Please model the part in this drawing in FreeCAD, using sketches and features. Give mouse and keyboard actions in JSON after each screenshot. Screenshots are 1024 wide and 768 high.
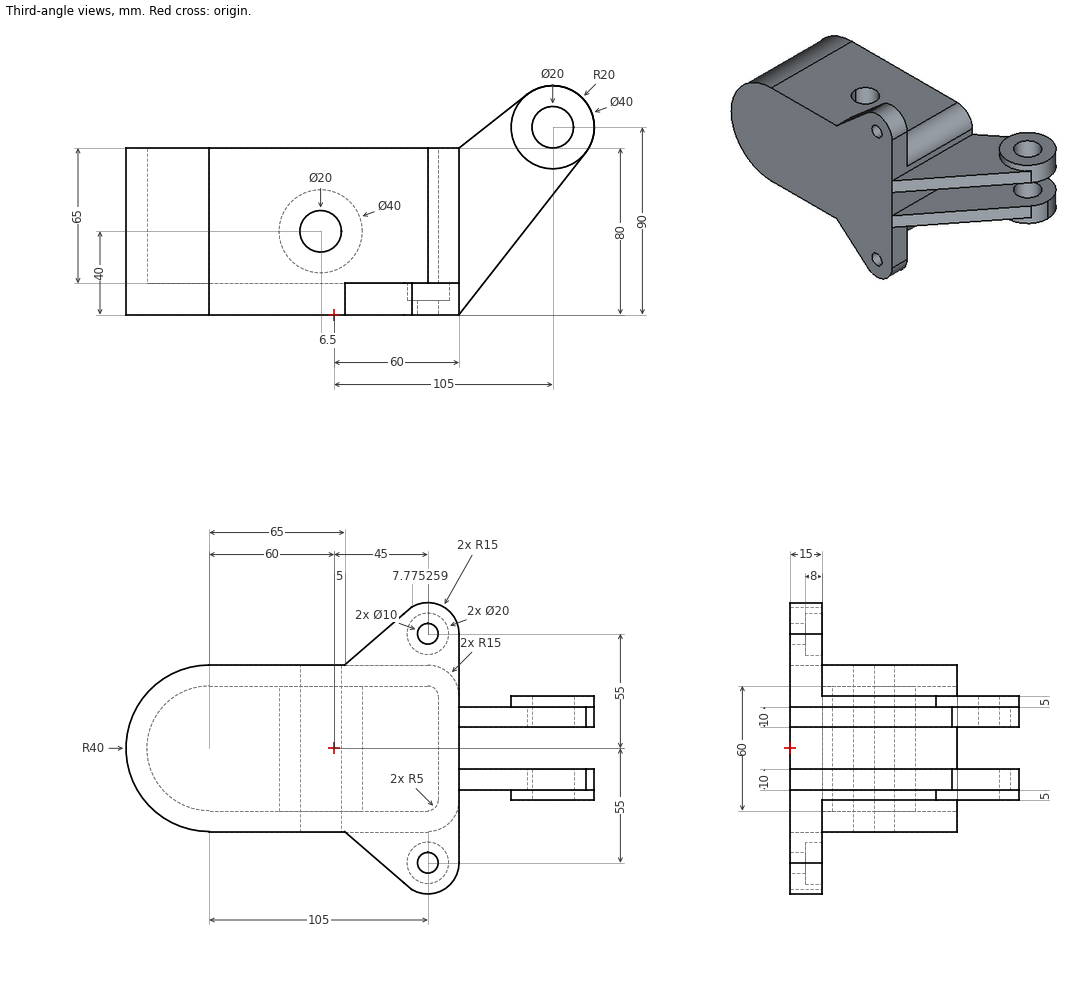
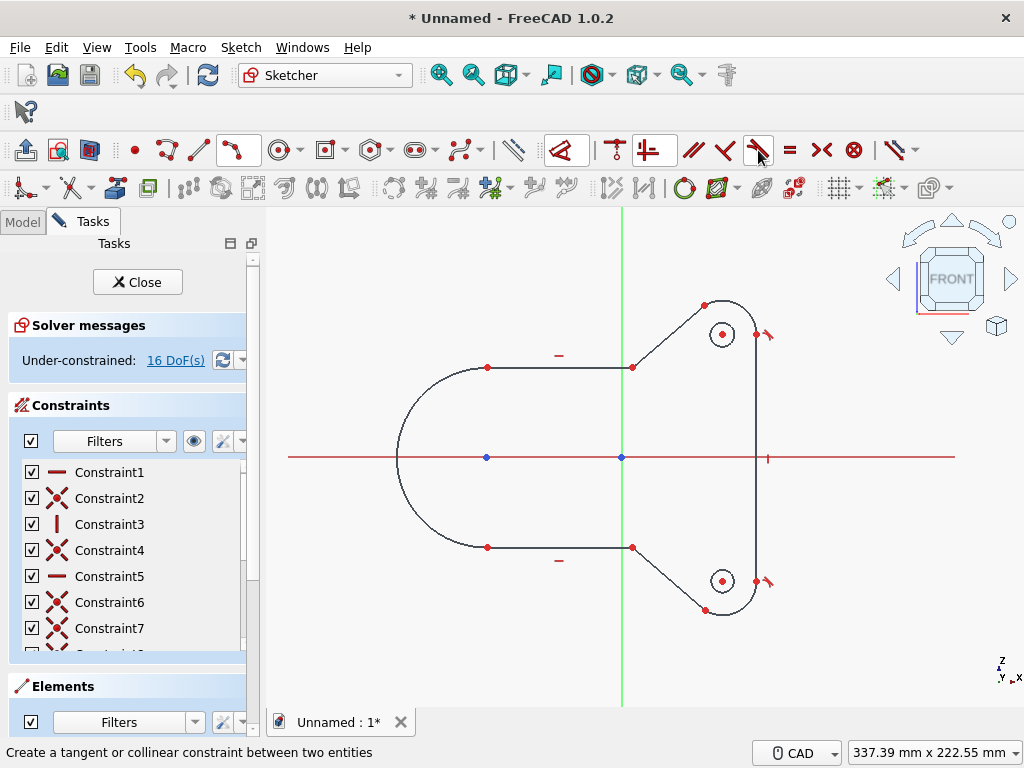
{"action": "left_click", "coordinate": [750, 315]}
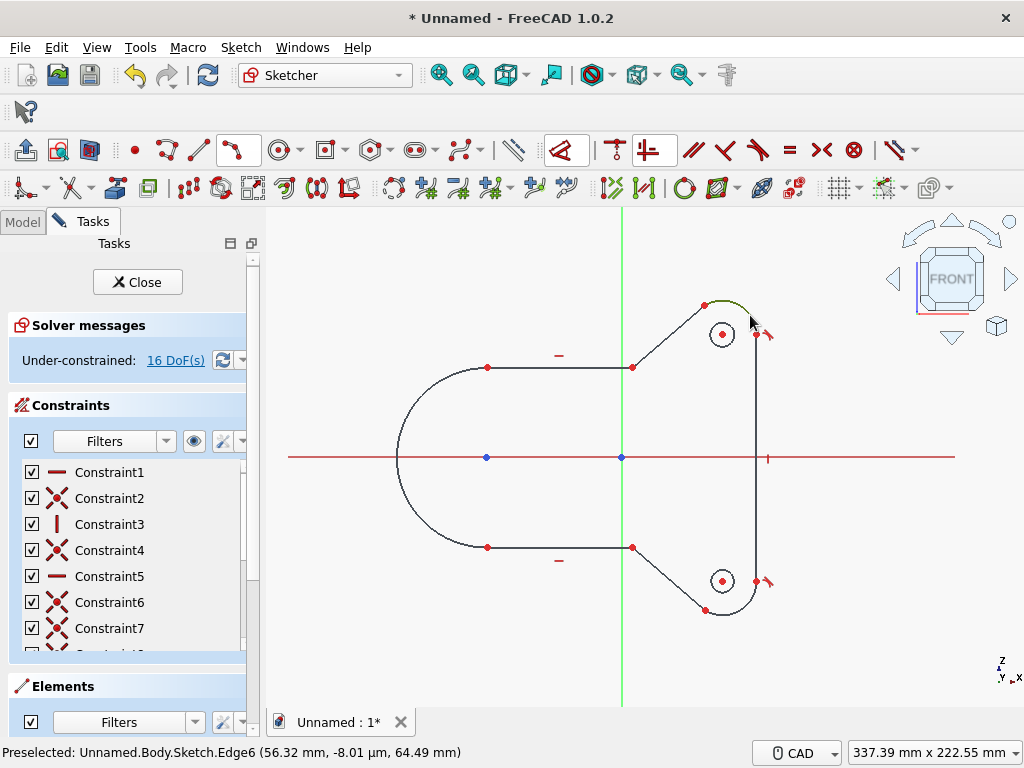
{"action": "left_click", "coordinate": [726, 615]}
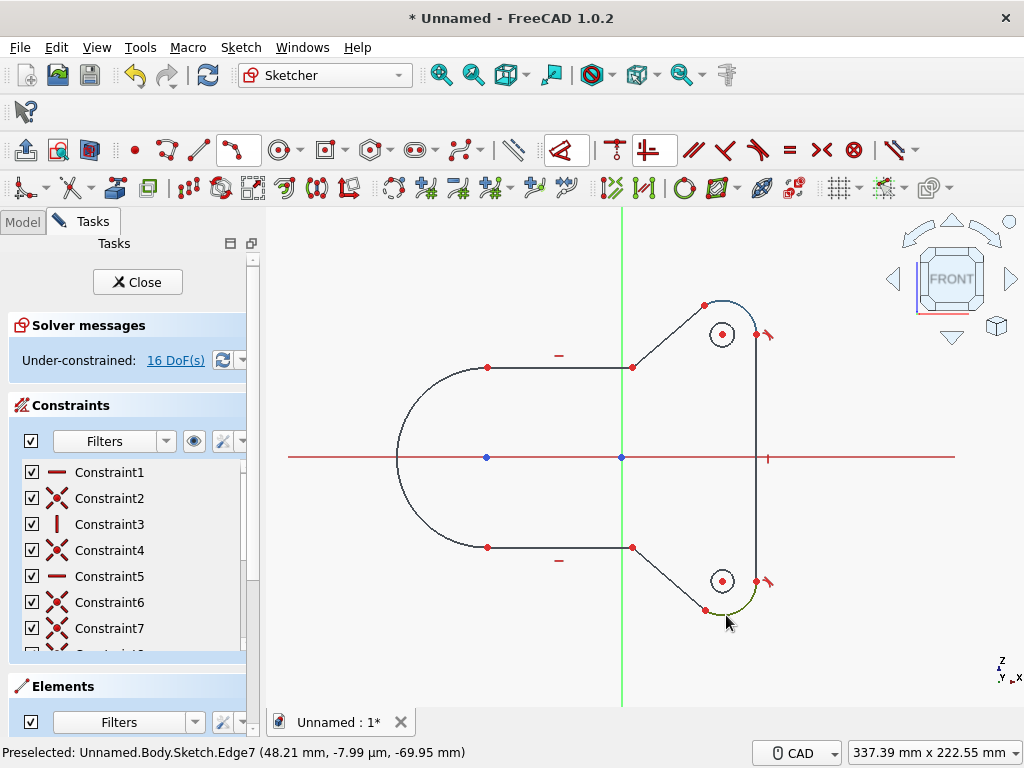
{"action": "left_click", "coordinate": [790, 150]}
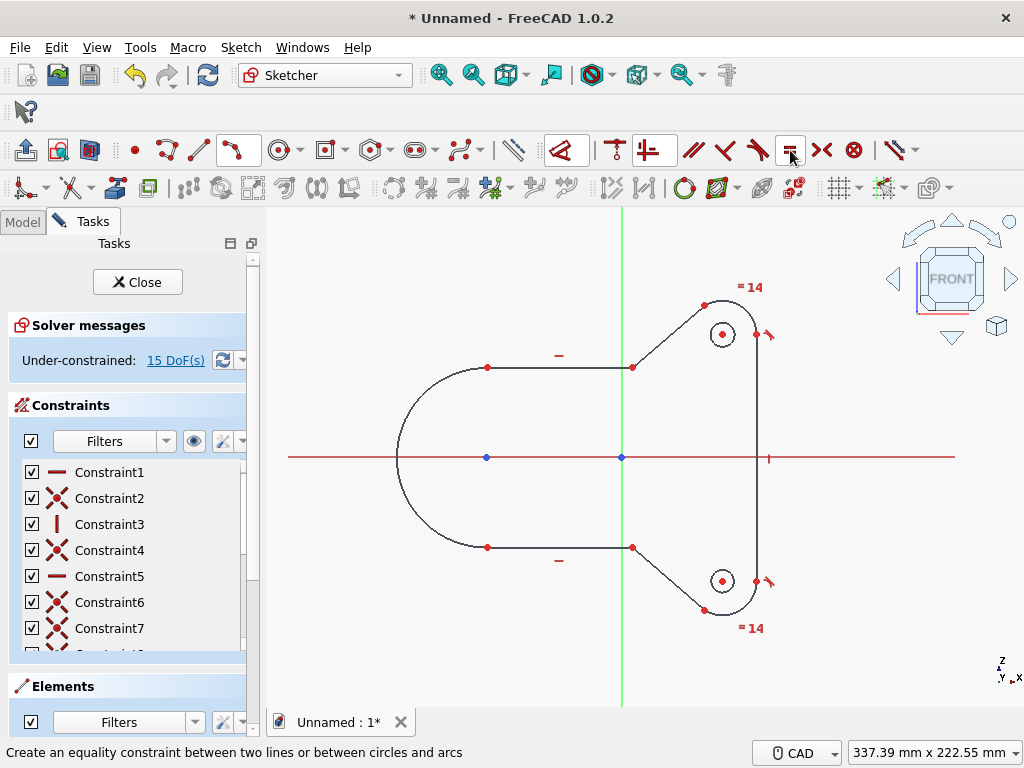
{"action": "left_click", "coordinate": [731, 326]}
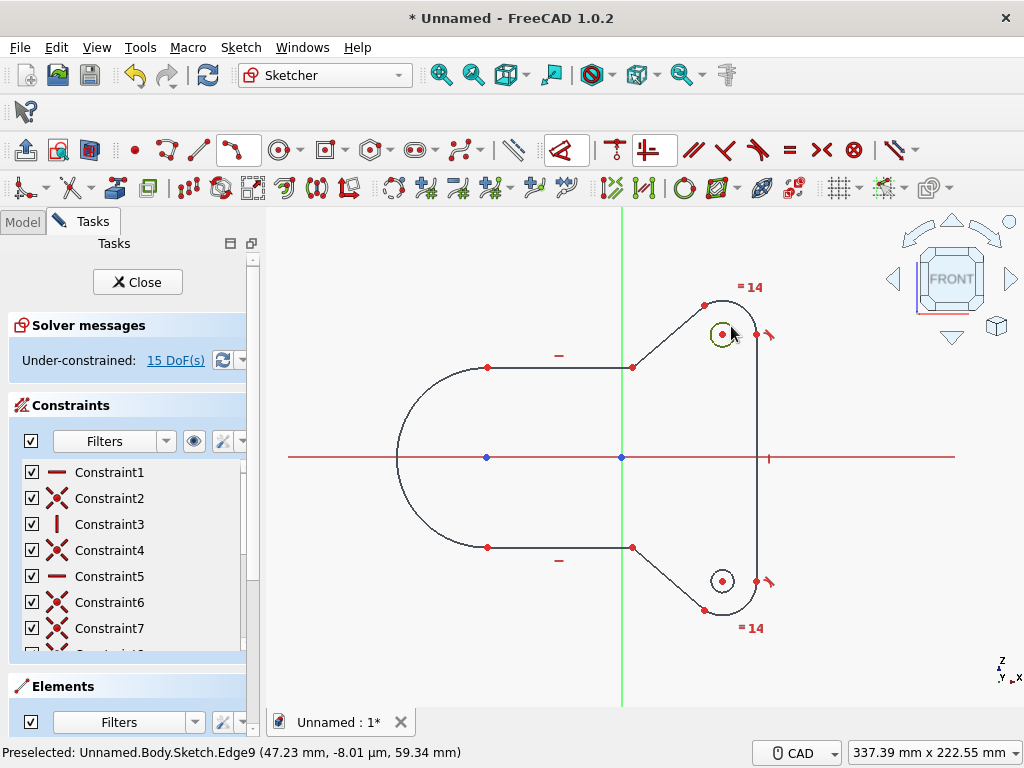
{"action": "scroll", "coordinate": [730, 573], "scroll_direction": "up", "scroll_amount": 2}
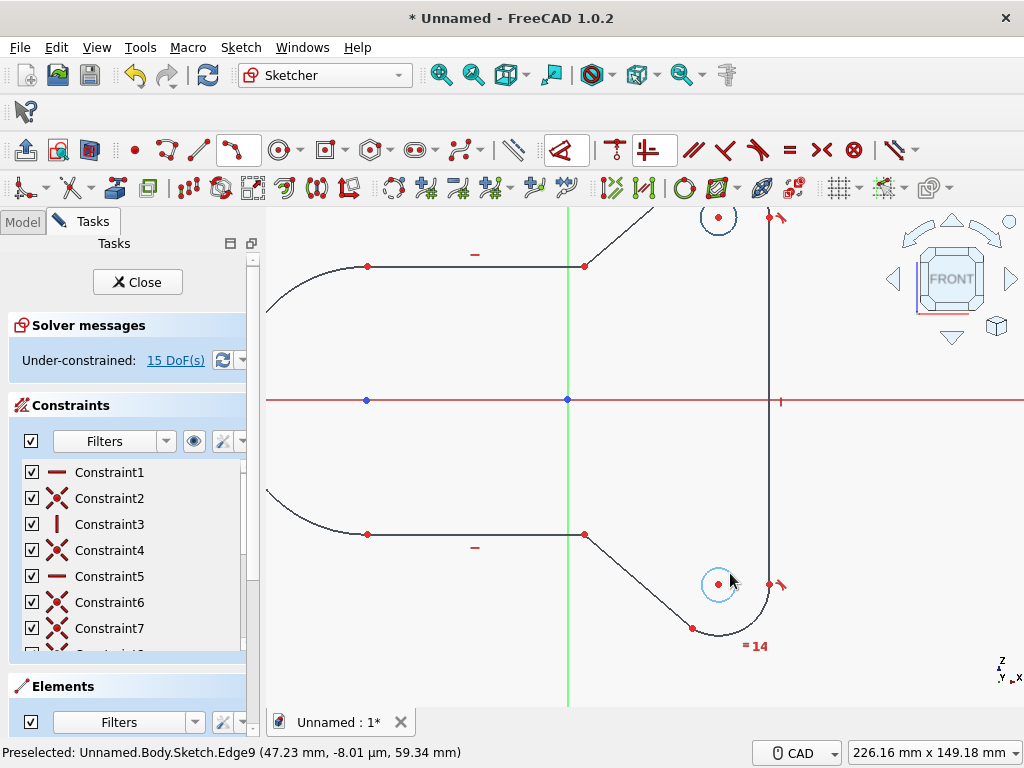
{"action": "left_click", "coordinate": [730, 573]}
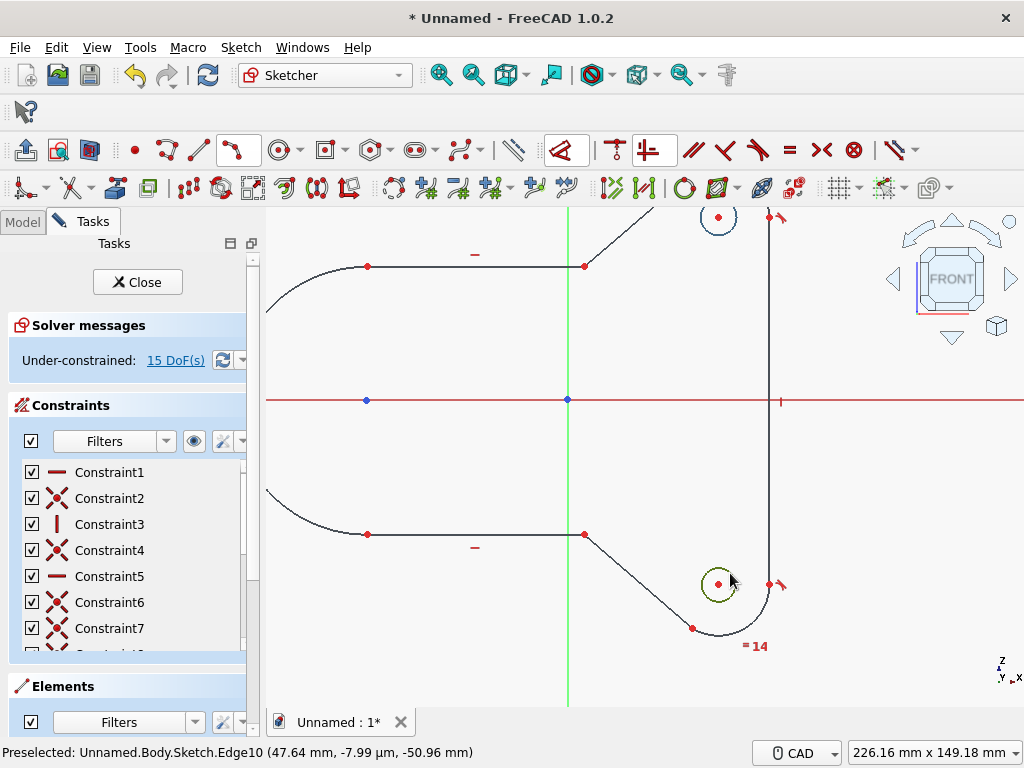
{"action": "left_click", "coordinate": [790, 150]}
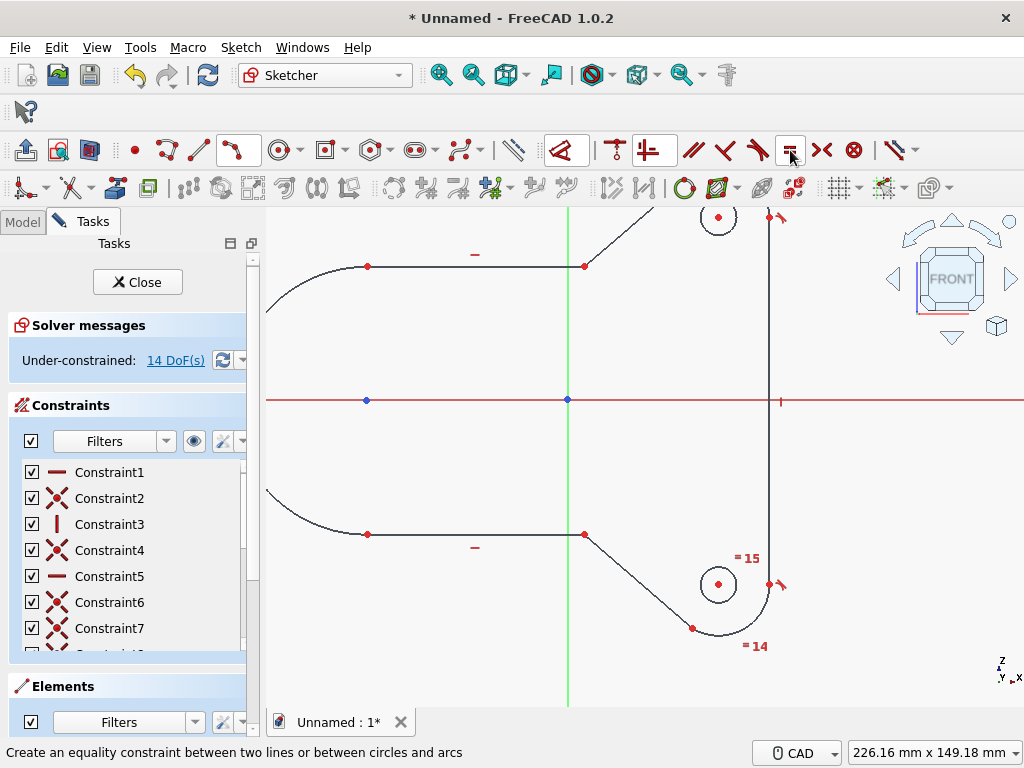
{"action": "left_click", "coordinate": [367, 401]}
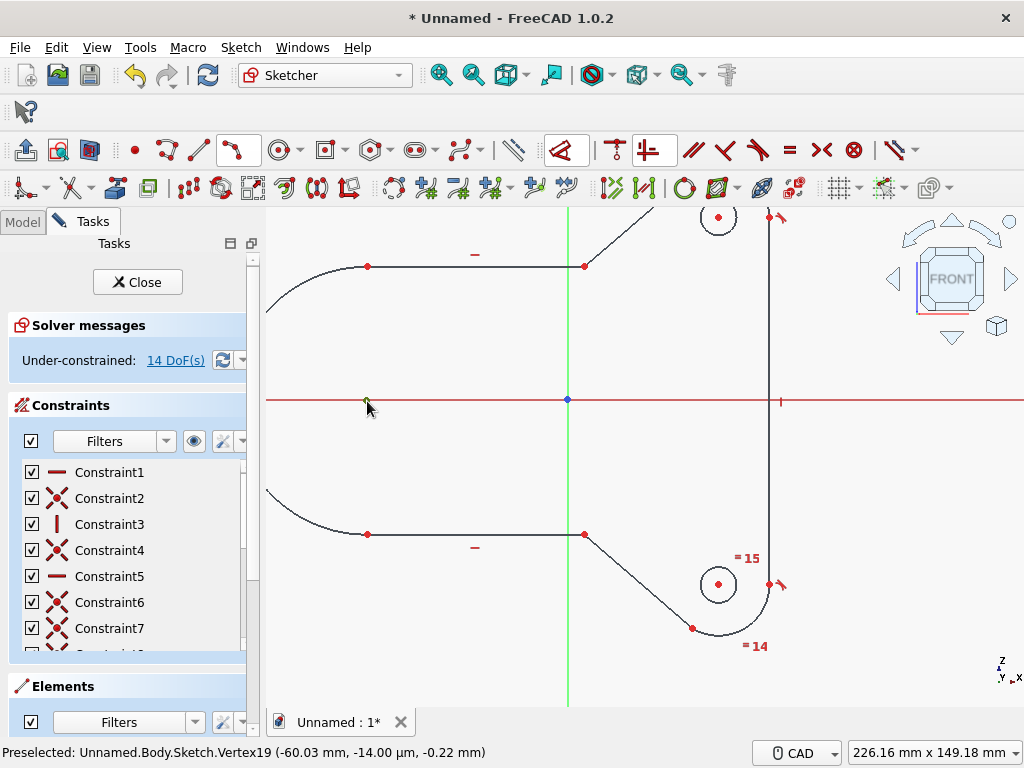
{"action": "left_click", "coordinate": [334, 400]}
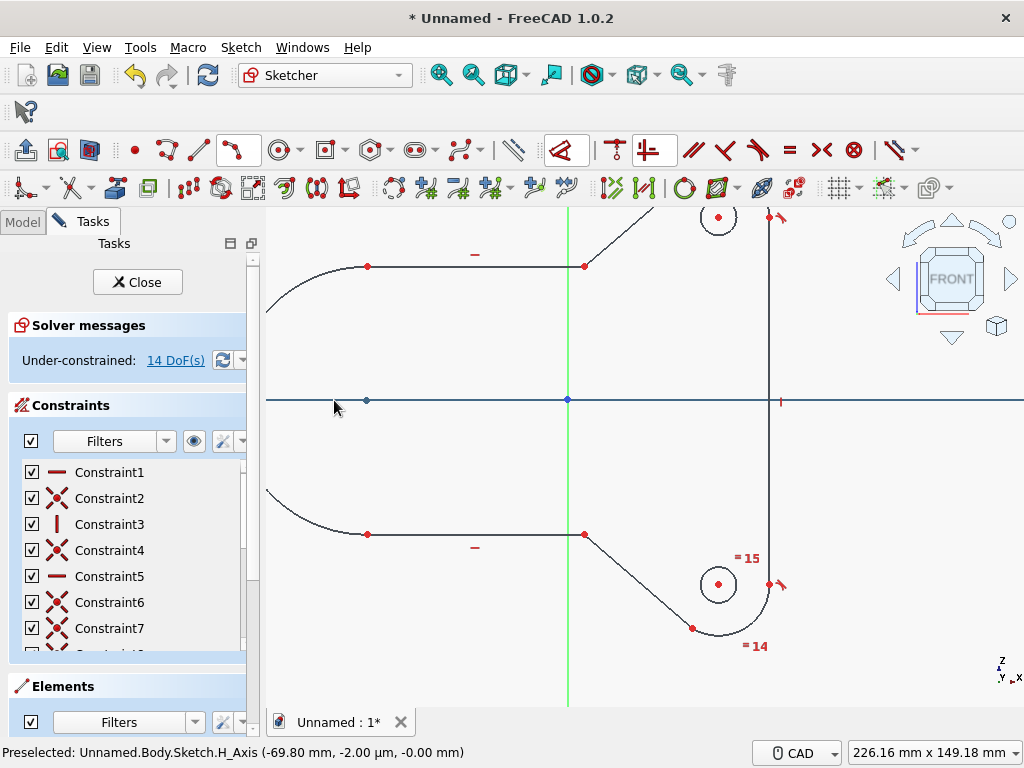
{"action": "left_click", "coordinate": [616, 150]}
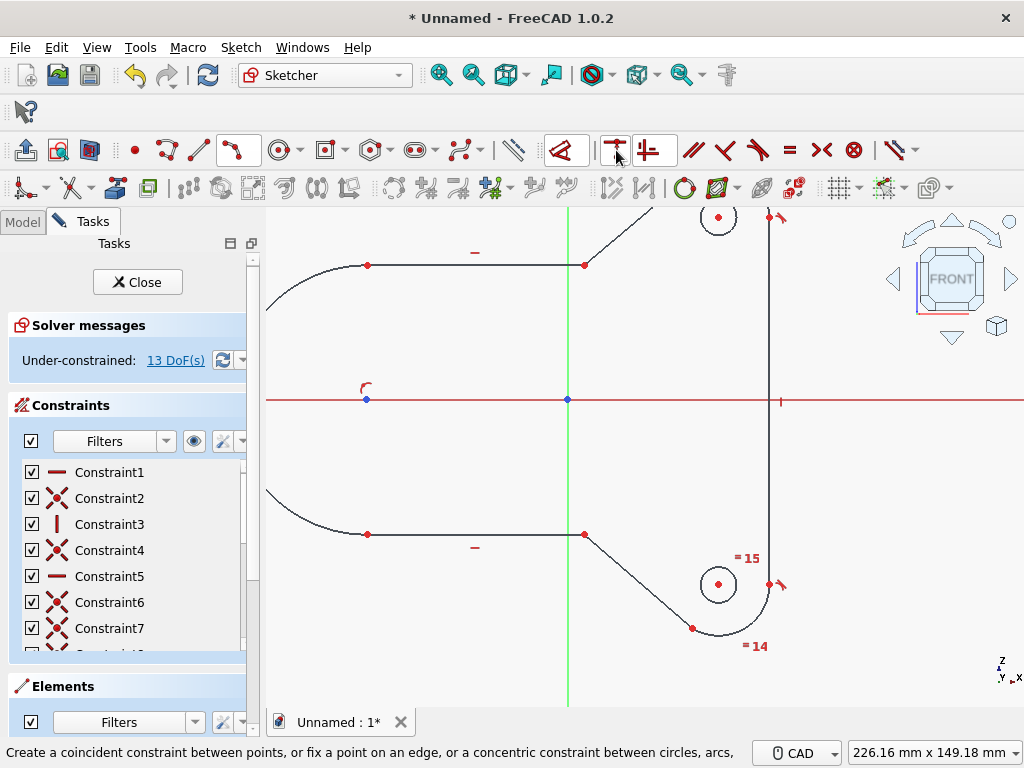
{"action": "scroll", "coordinate": [730, 573], "scroll_direction": "down", "scroll_amount": 2}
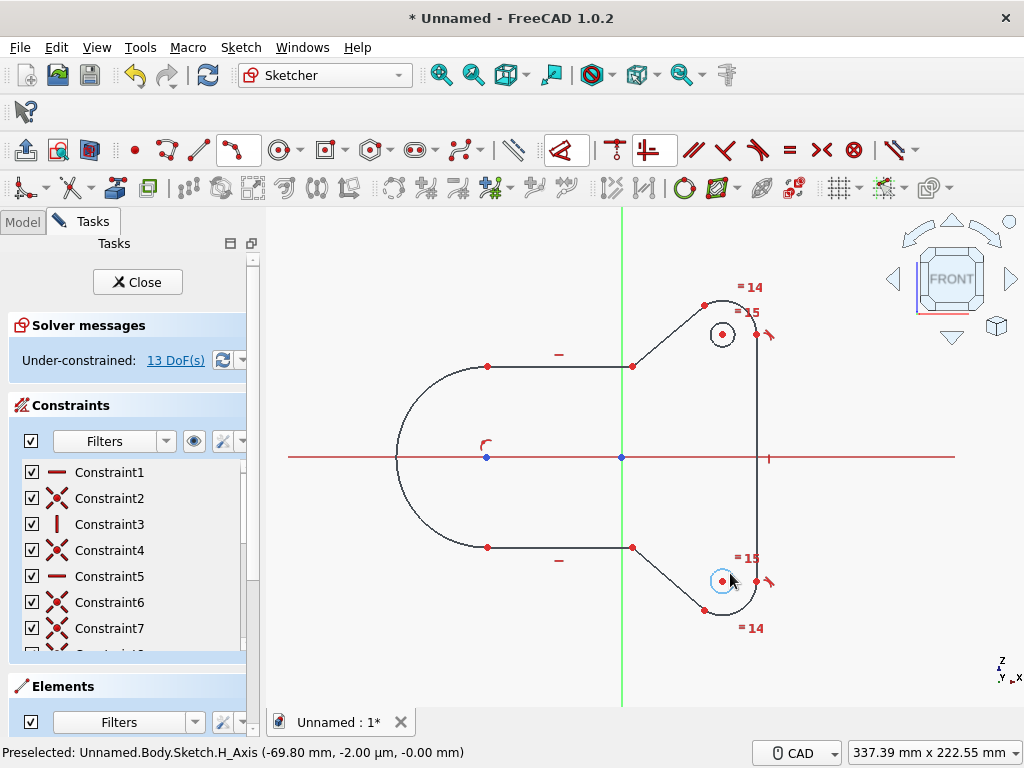
{"action": "left_click", "coordinate": [726, 301]}